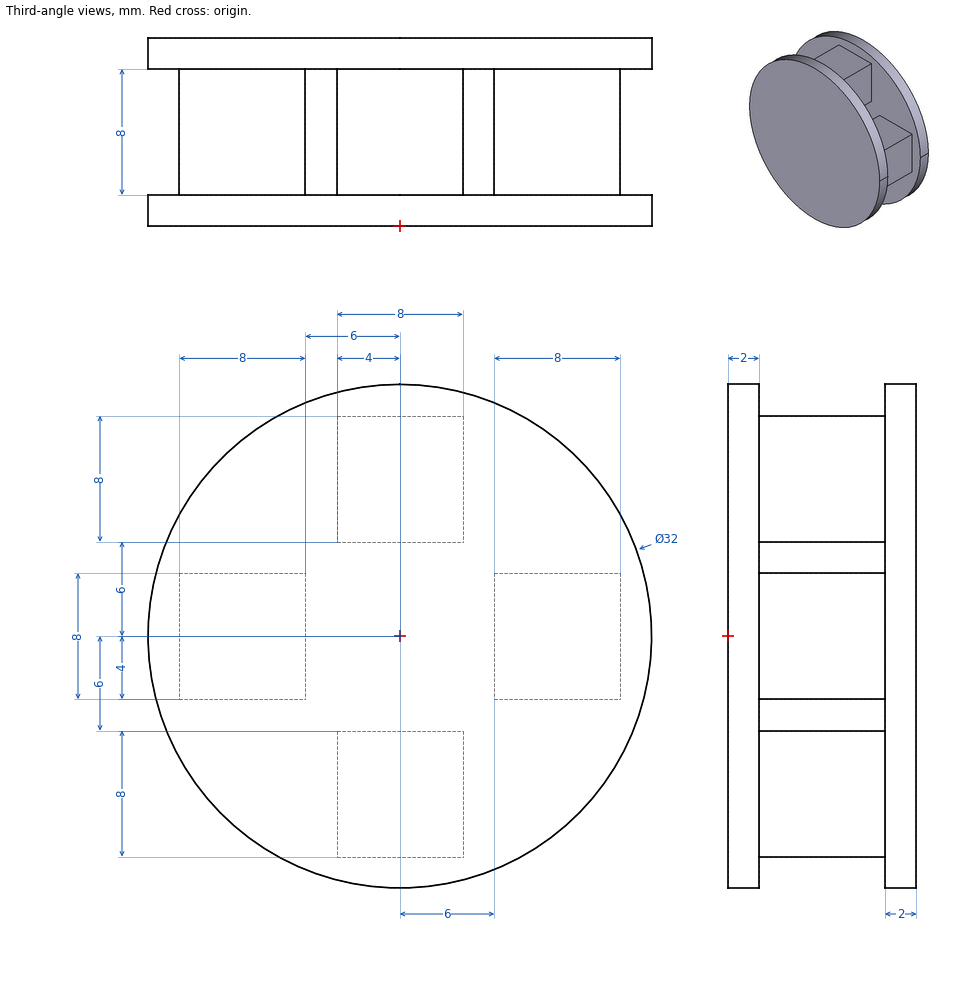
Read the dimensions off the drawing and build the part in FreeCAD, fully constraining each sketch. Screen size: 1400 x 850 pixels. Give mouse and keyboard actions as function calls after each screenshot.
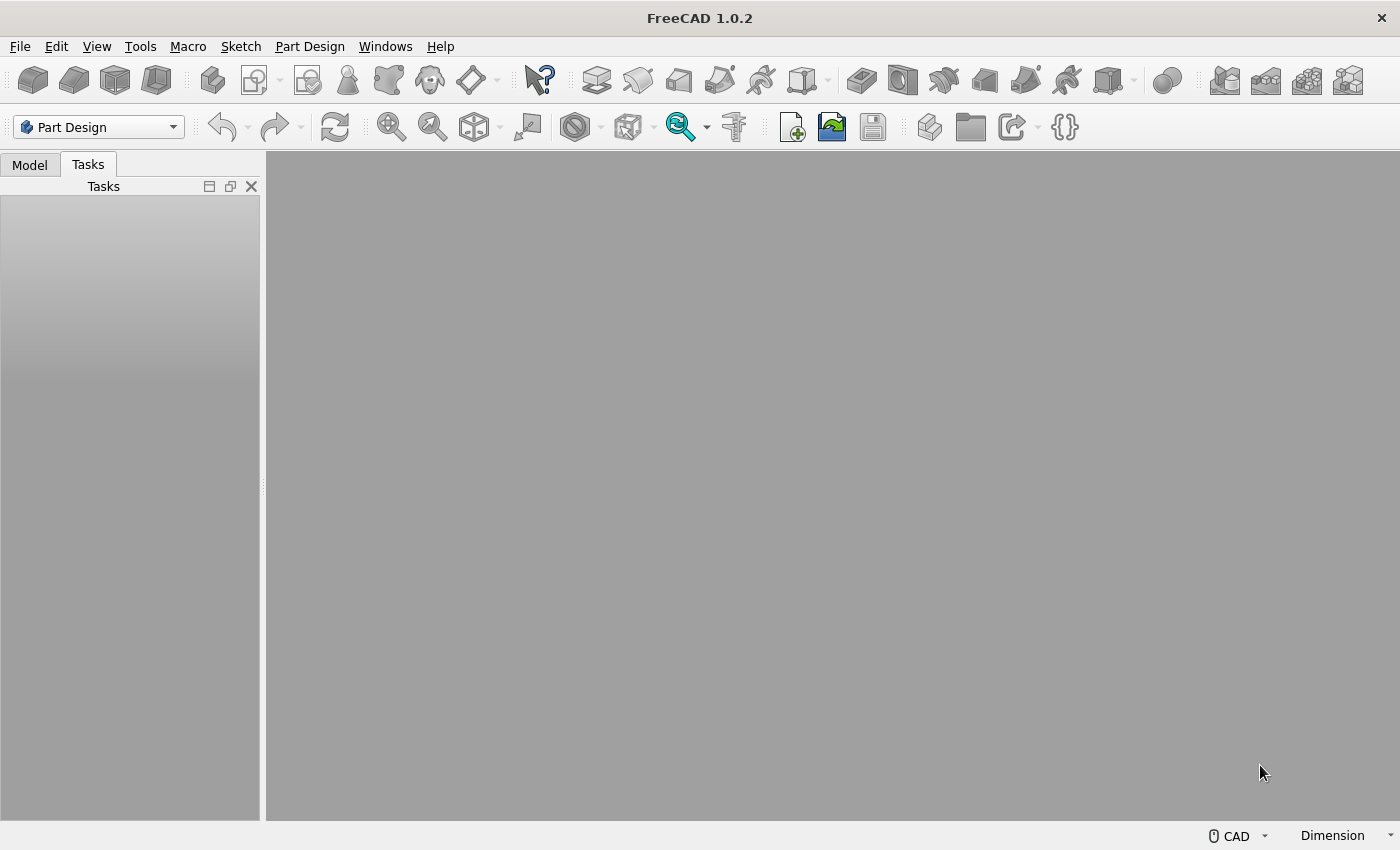
key(ctrl+n)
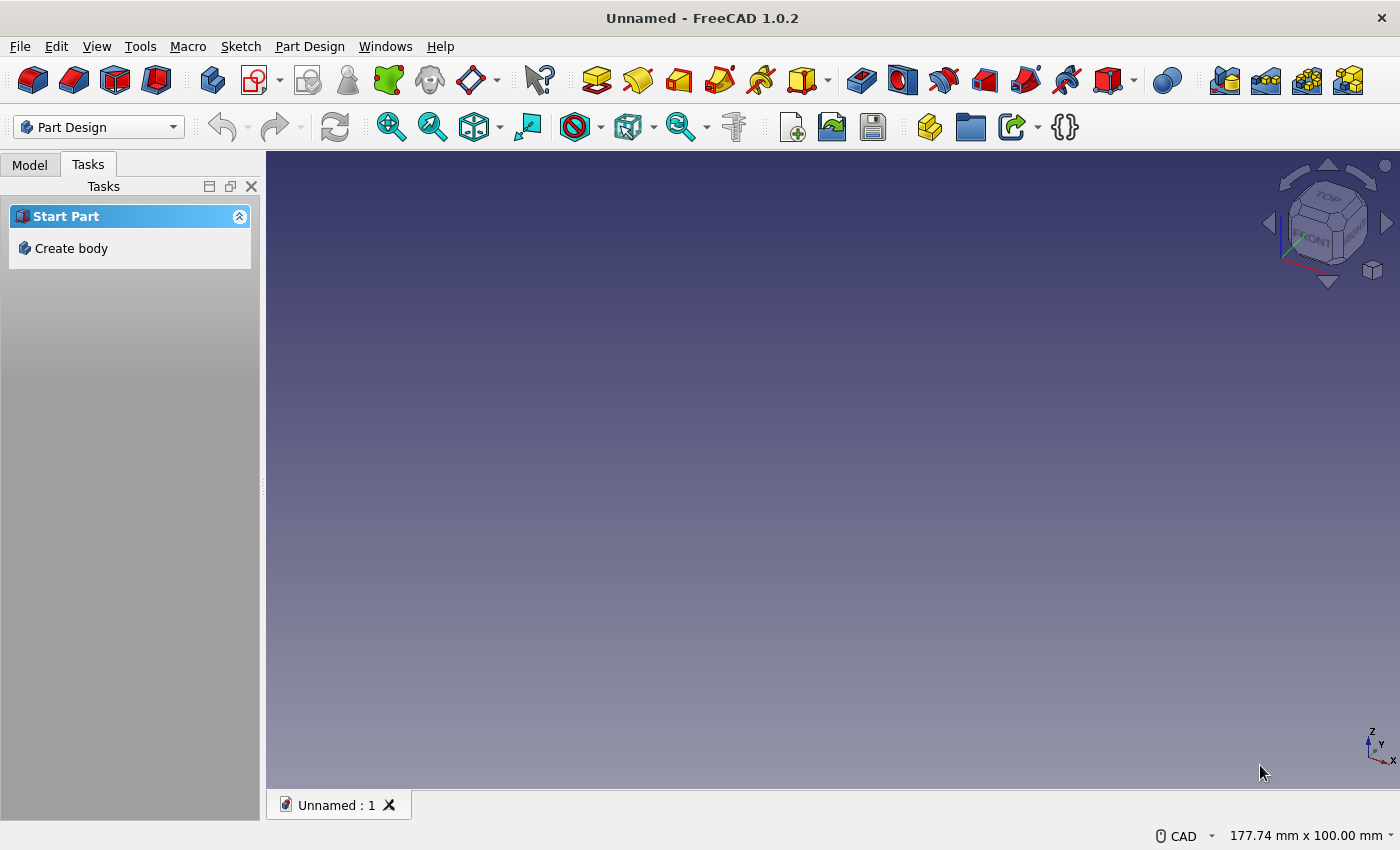
click(254, 80)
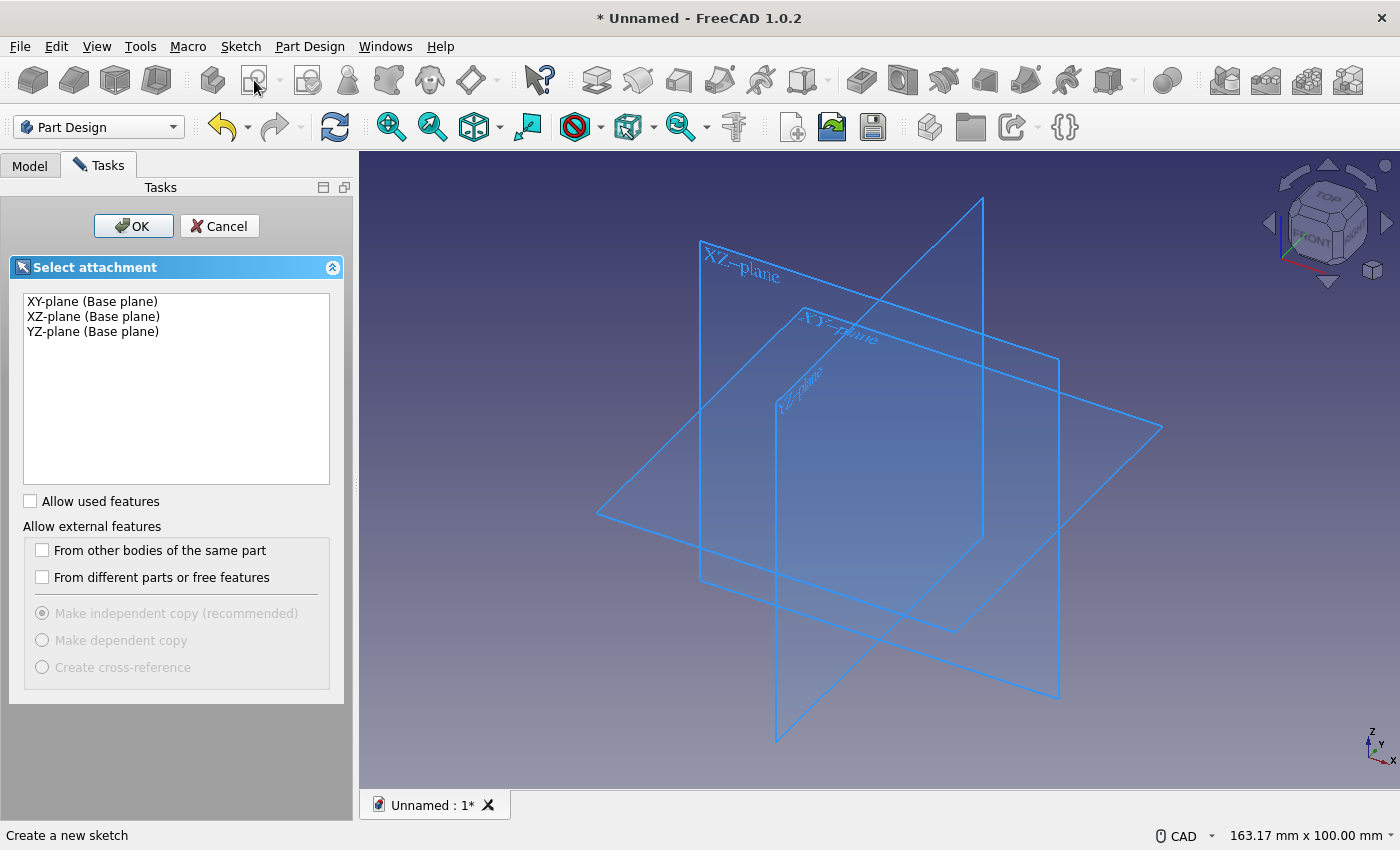
click(84, 316)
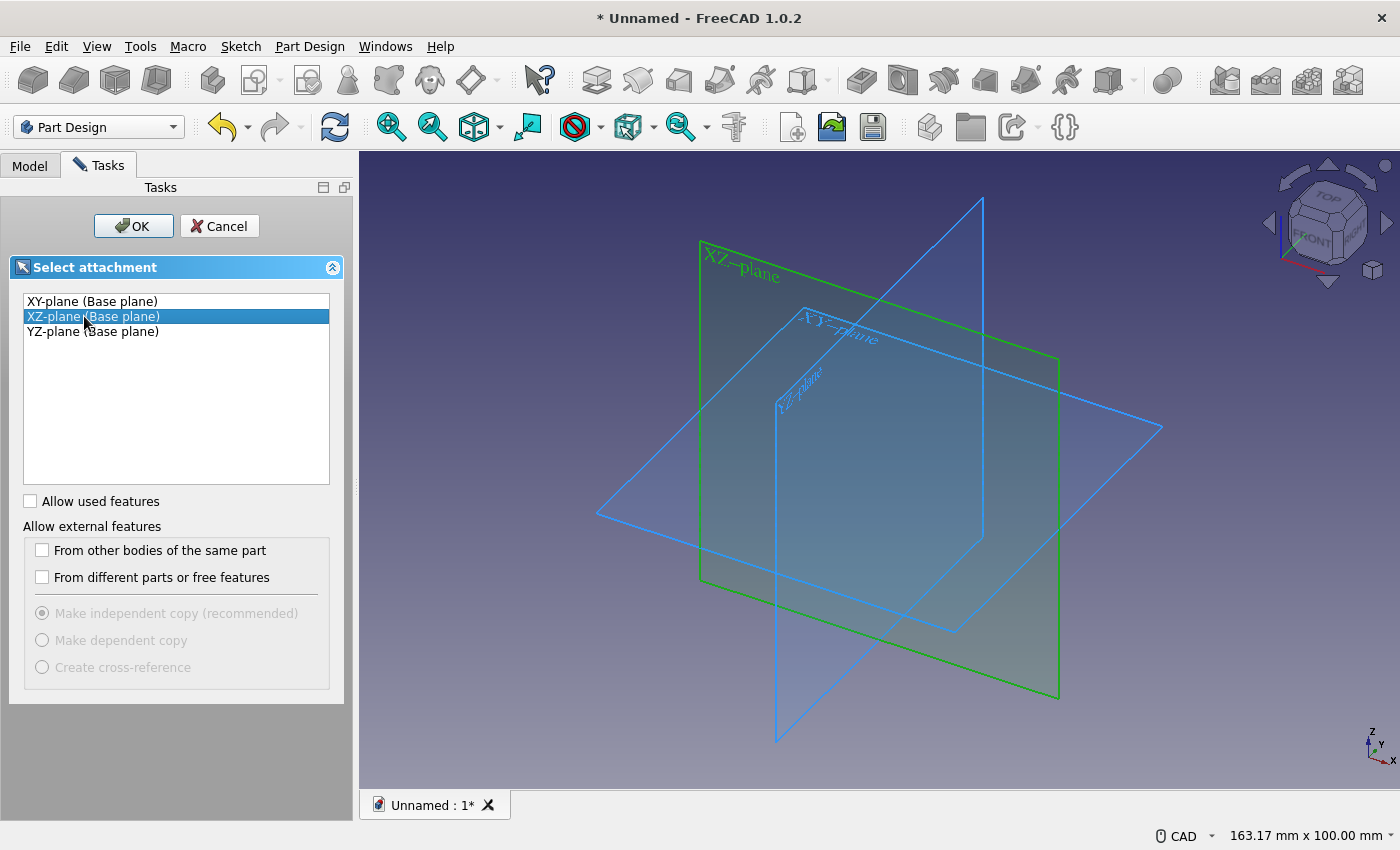
click(134, 226)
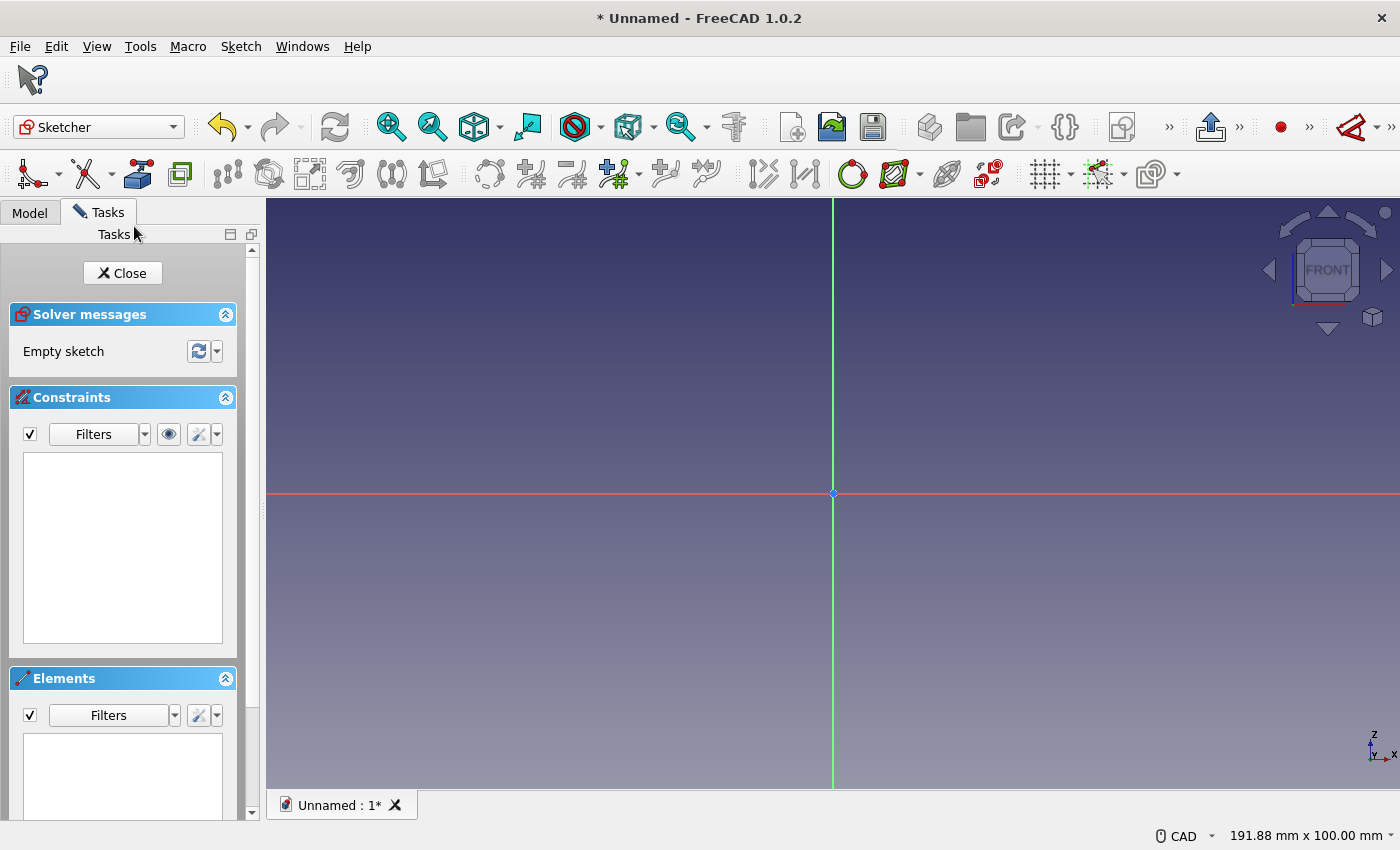
scroll(916, 494, up, 3)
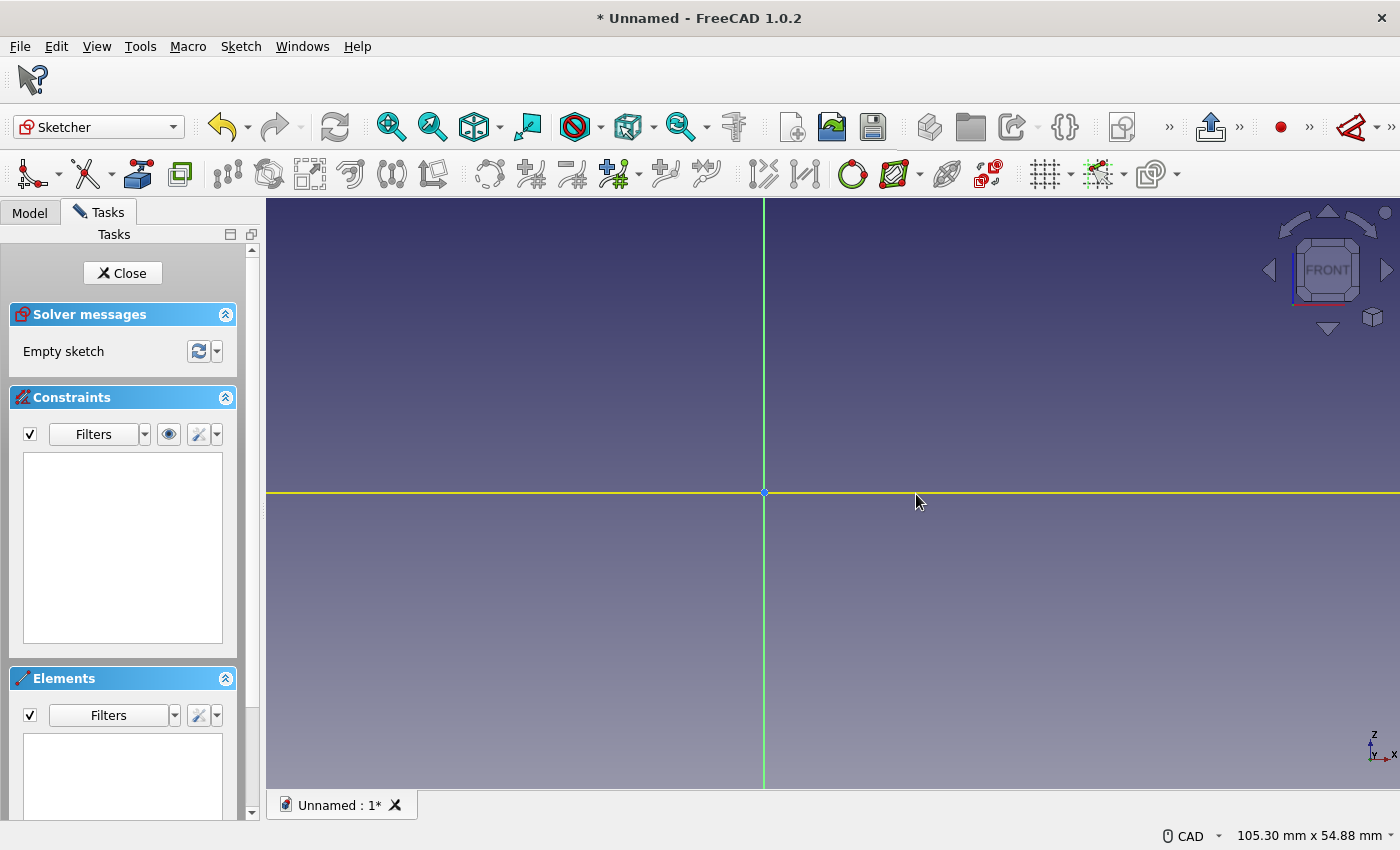
key(g)
key(c)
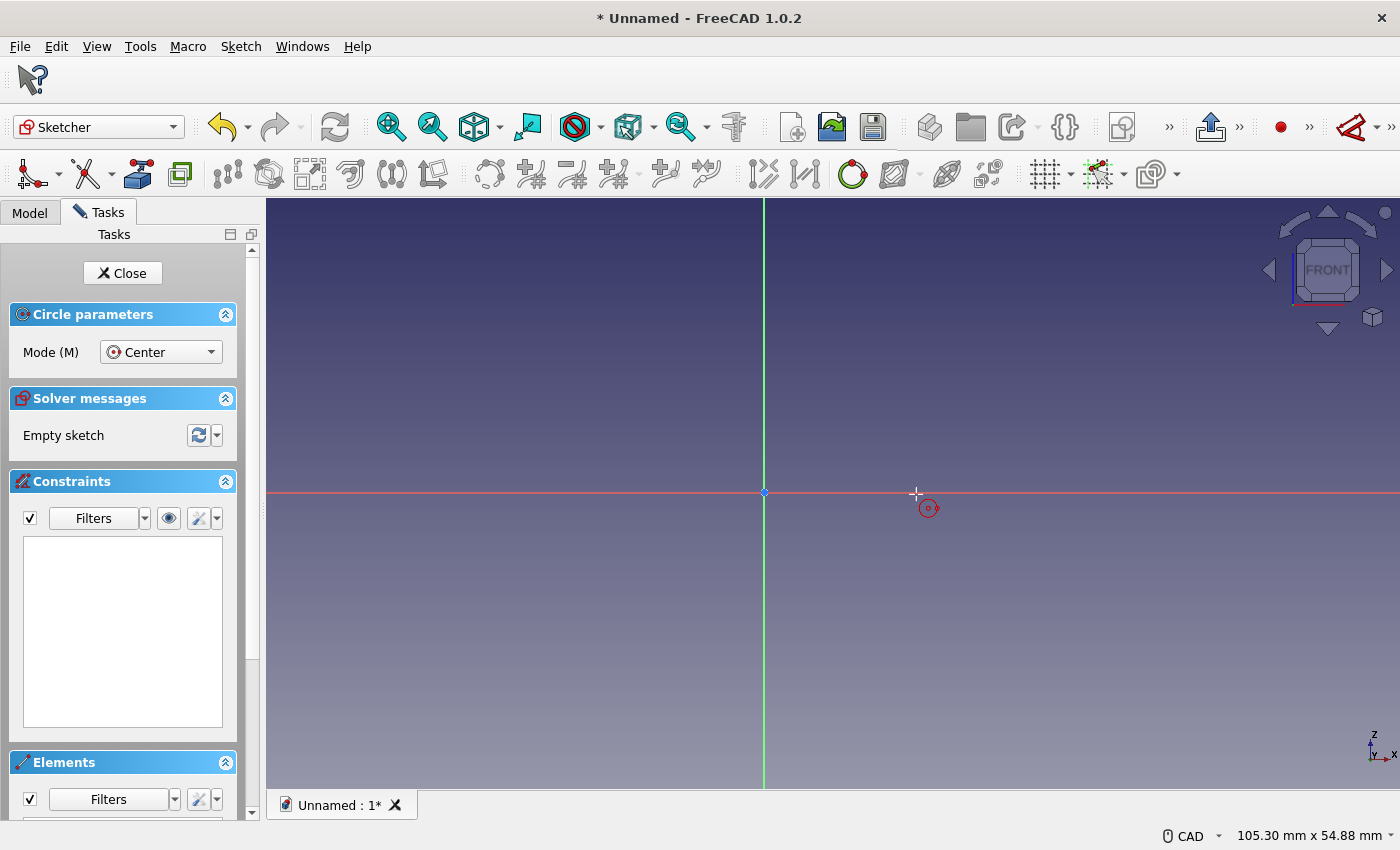
click(764, 493)
click(886, 371)
key(Escape)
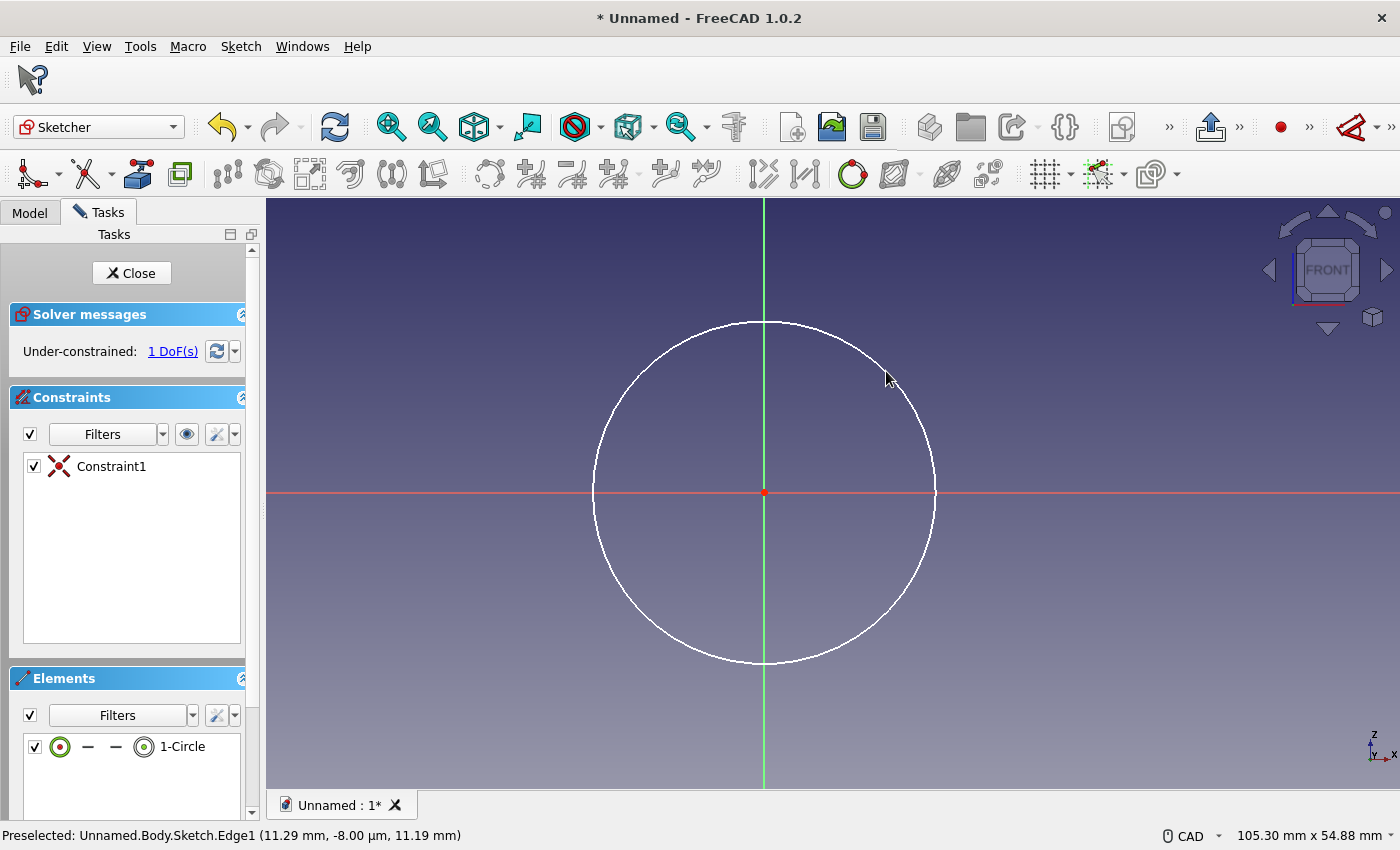
key(d)